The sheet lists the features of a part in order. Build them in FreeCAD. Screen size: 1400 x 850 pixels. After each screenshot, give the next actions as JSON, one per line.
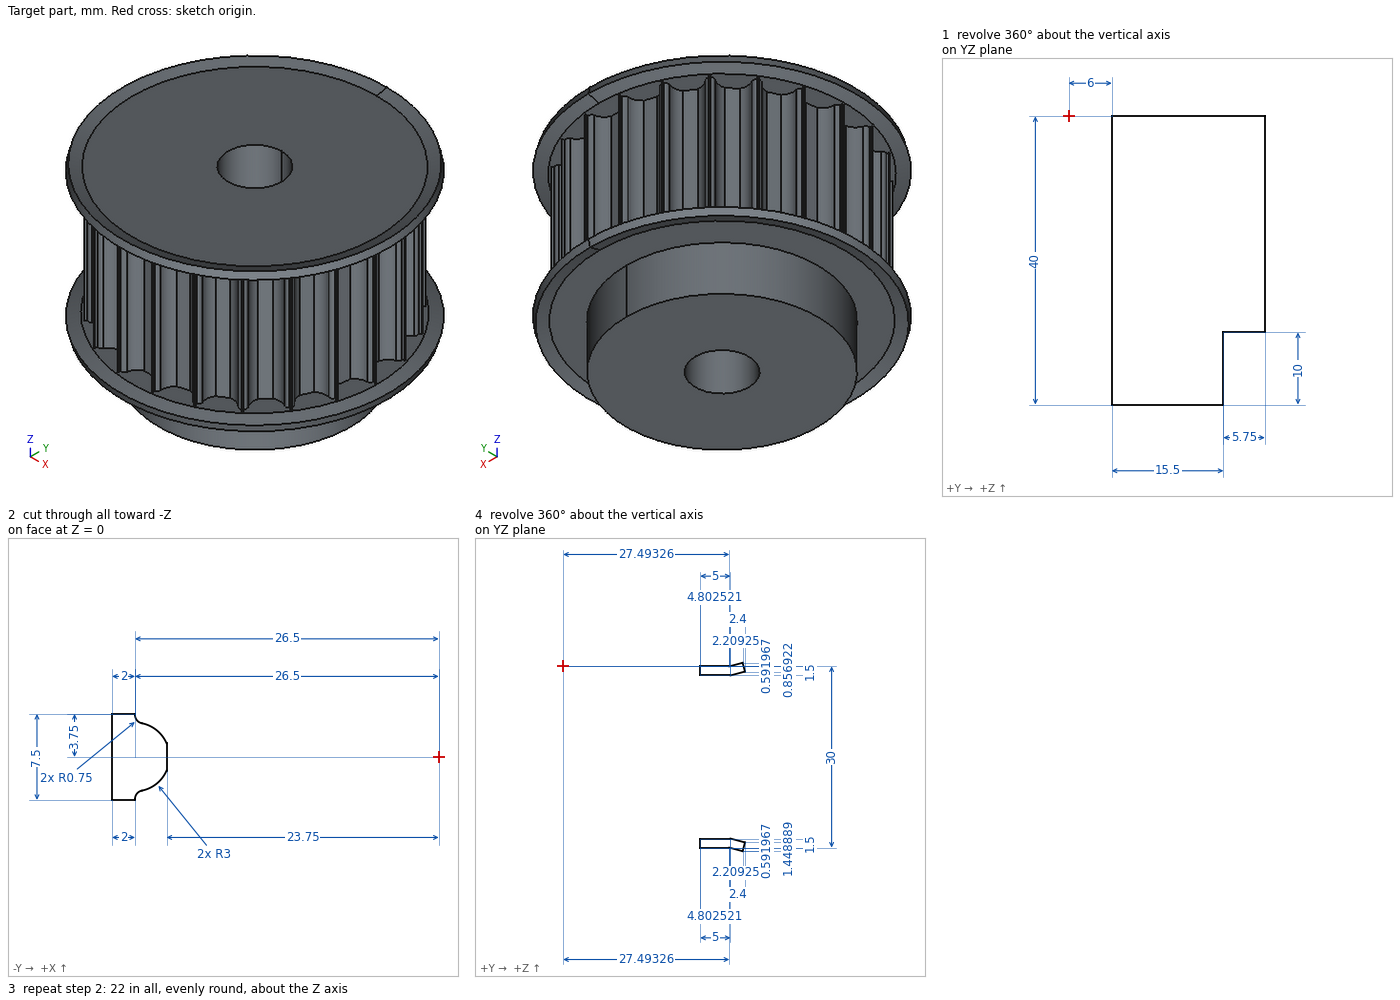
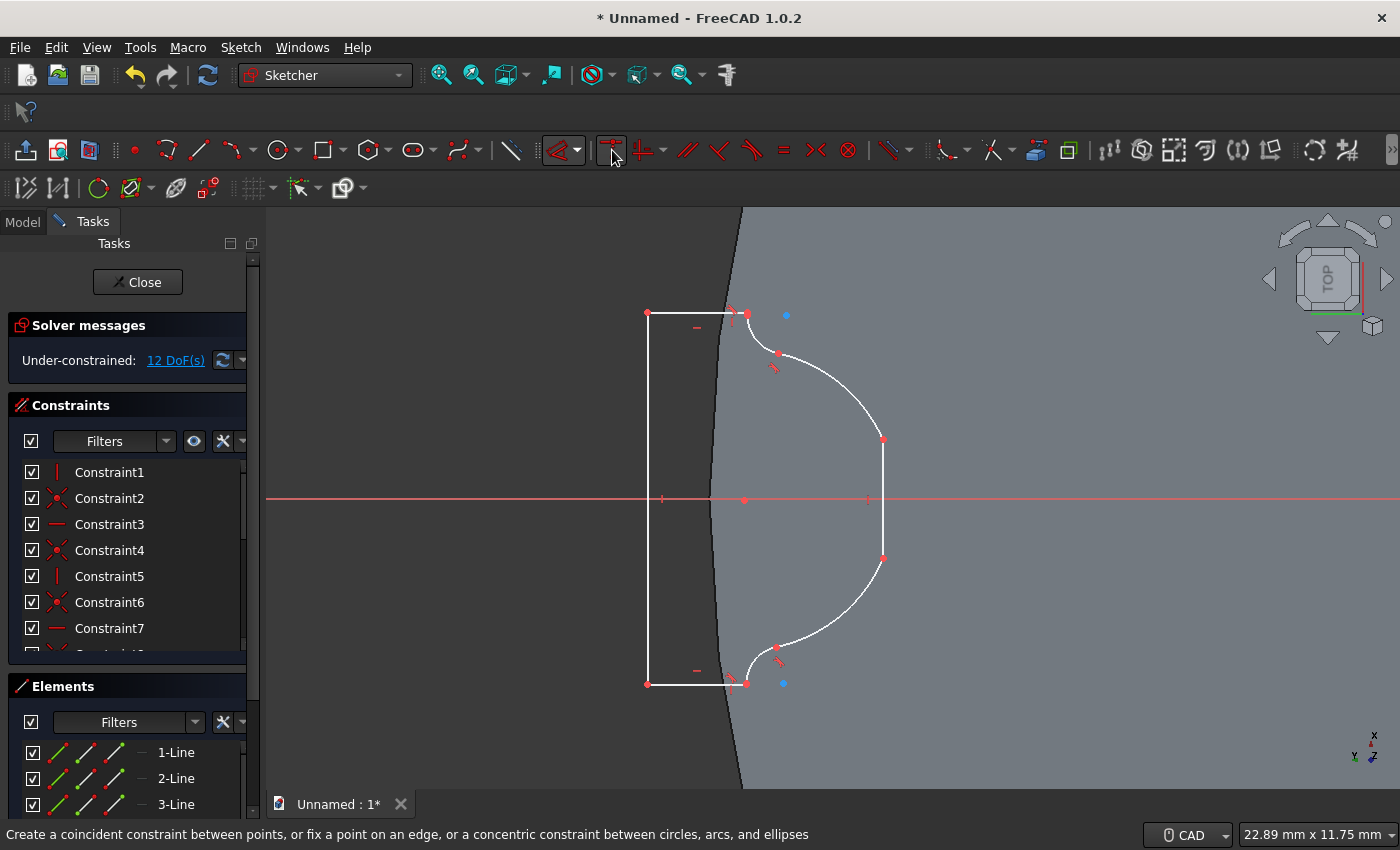
{"action": "left_click", "coordinate": [817, 632]}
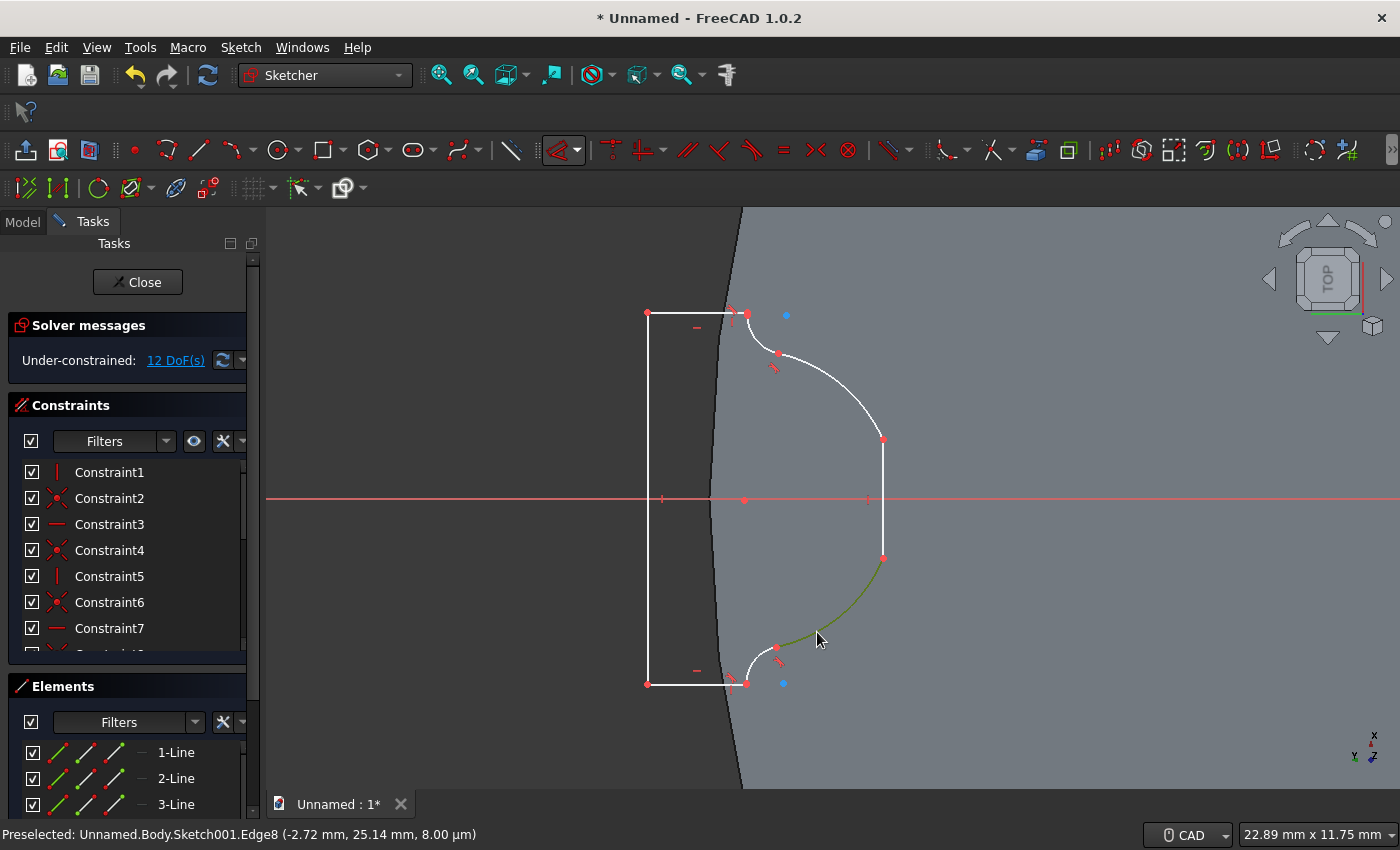
{"action": "left_click", "coordinate": [861, 404]}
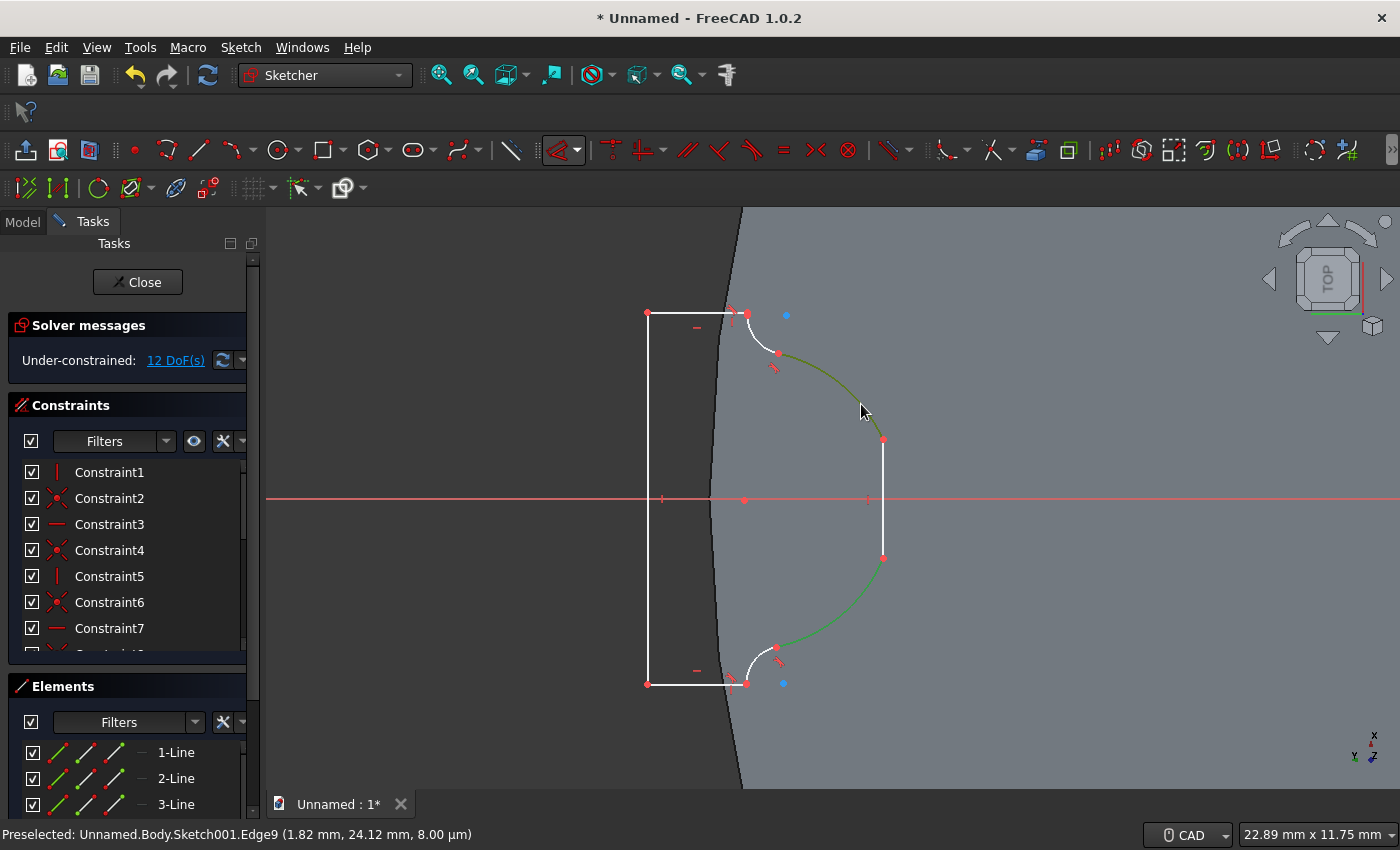
{"action": "left_click", "coordinate": [784, 150]}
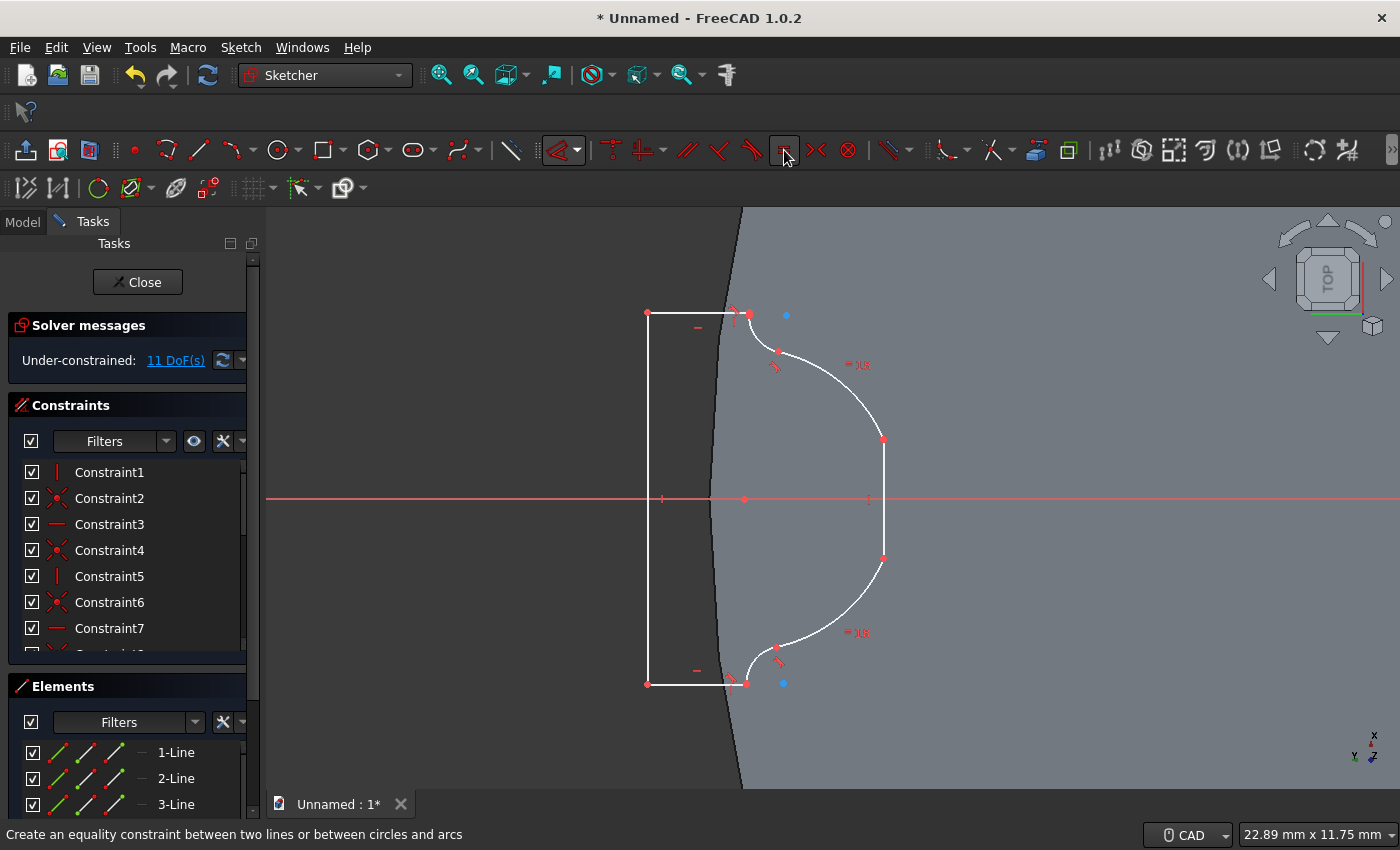
{"action": "left_click", "coordinate": [762, 653]}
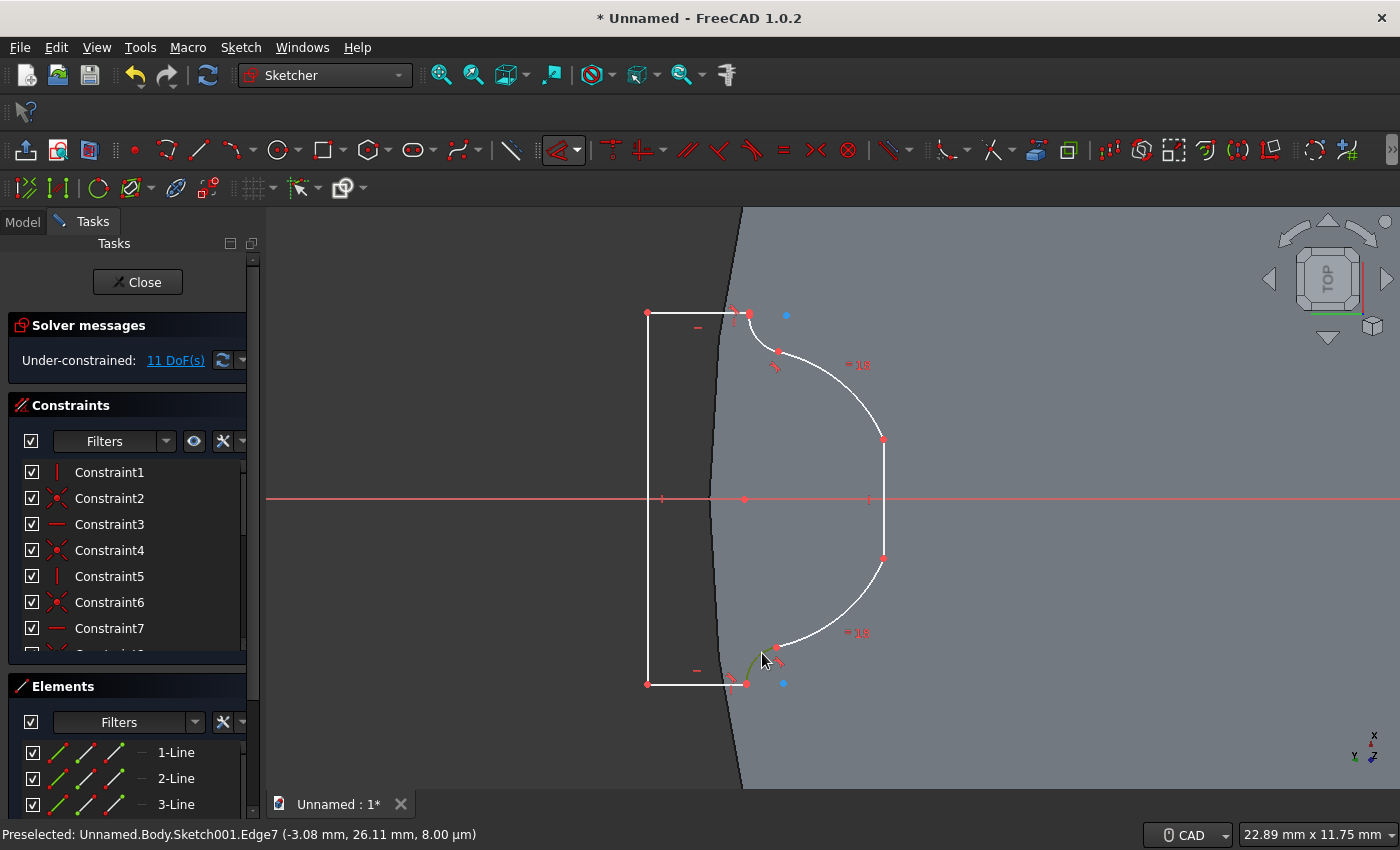
{"action": "left_click", "coordinate": [752, 330]}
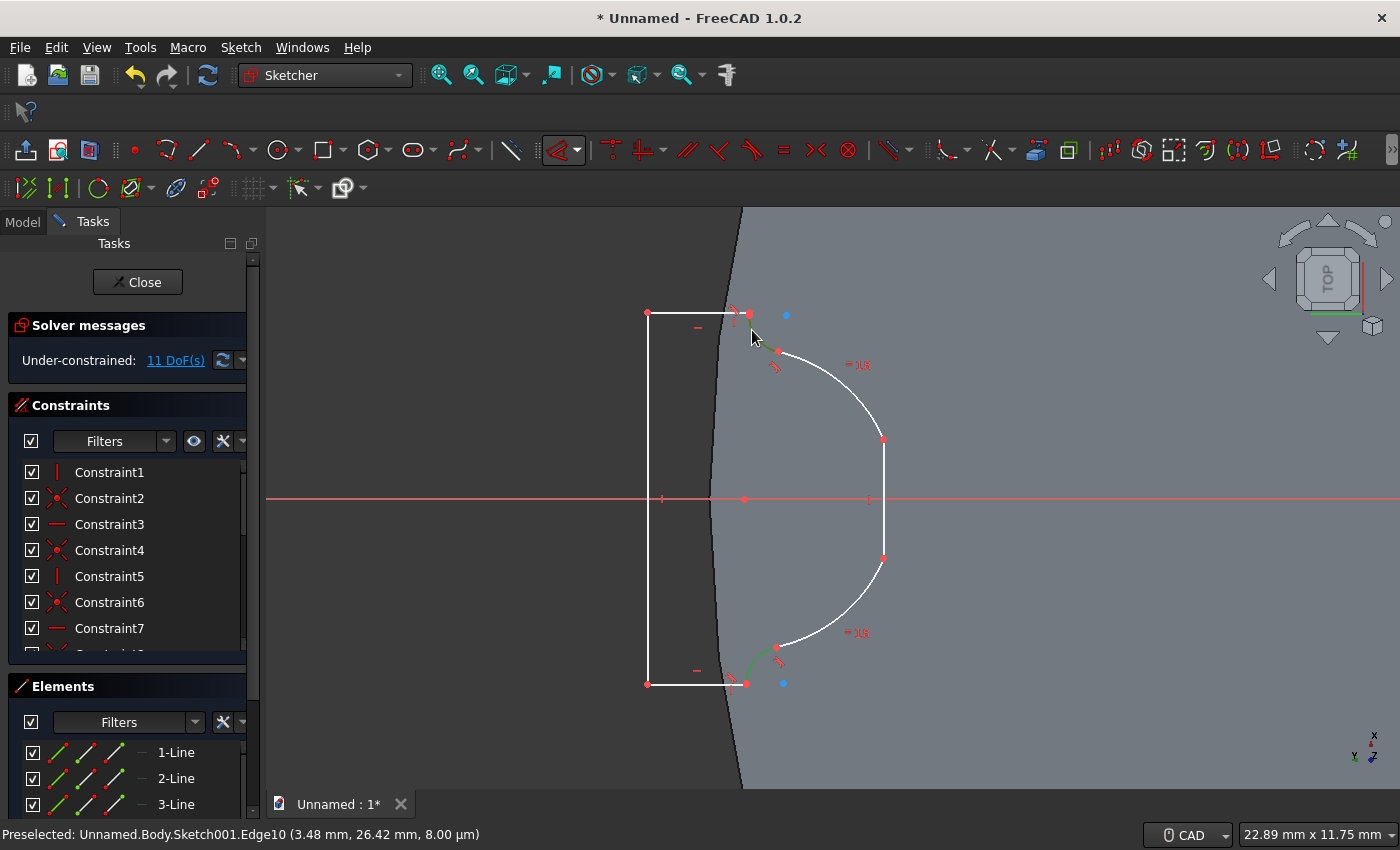
{"action": "left_click", "coordinate": [784, 150]}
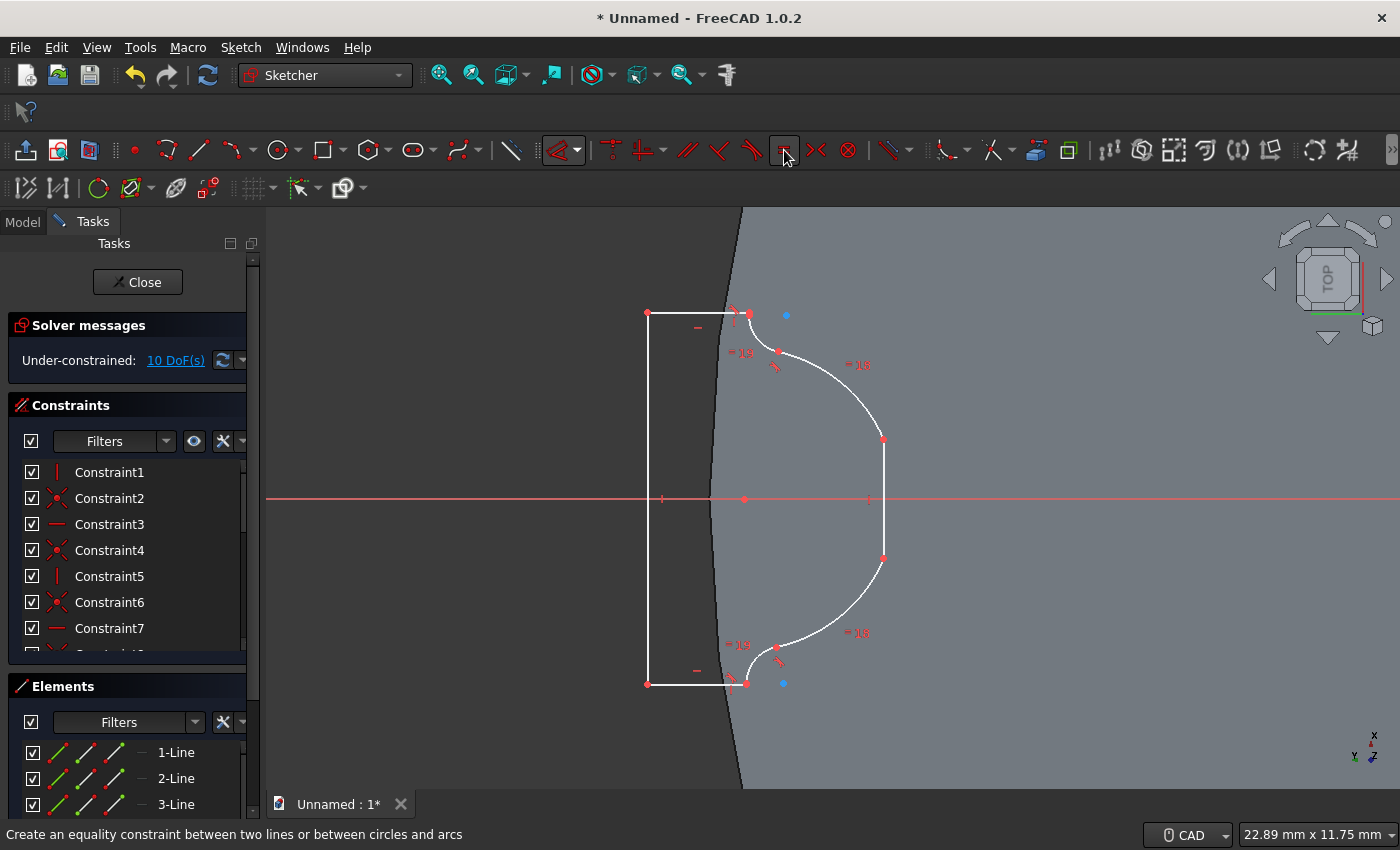
{"action": "left_click", "coordinate": [745, 499]}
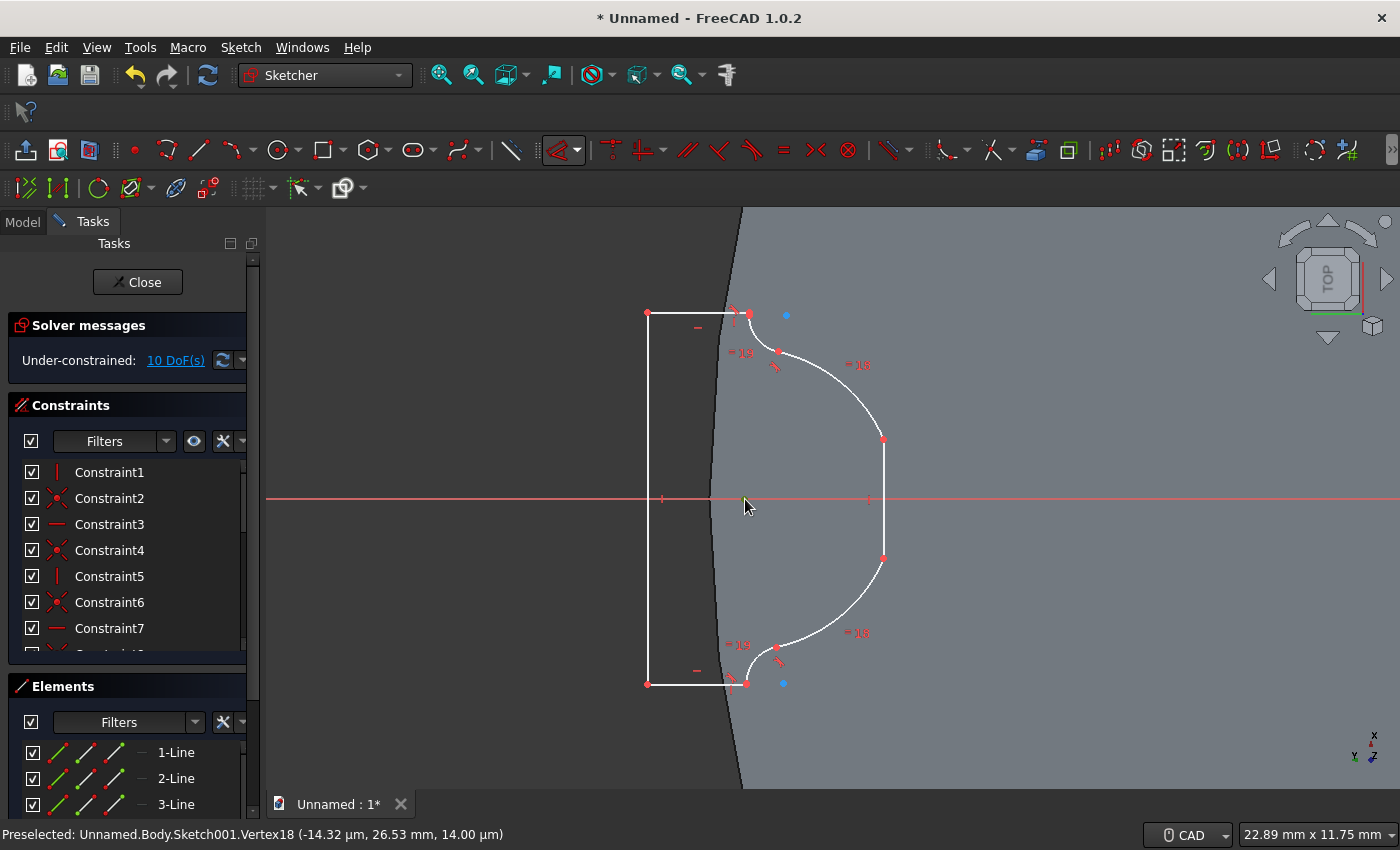
{"action": "left_click", "coordinate": [361, 499]}